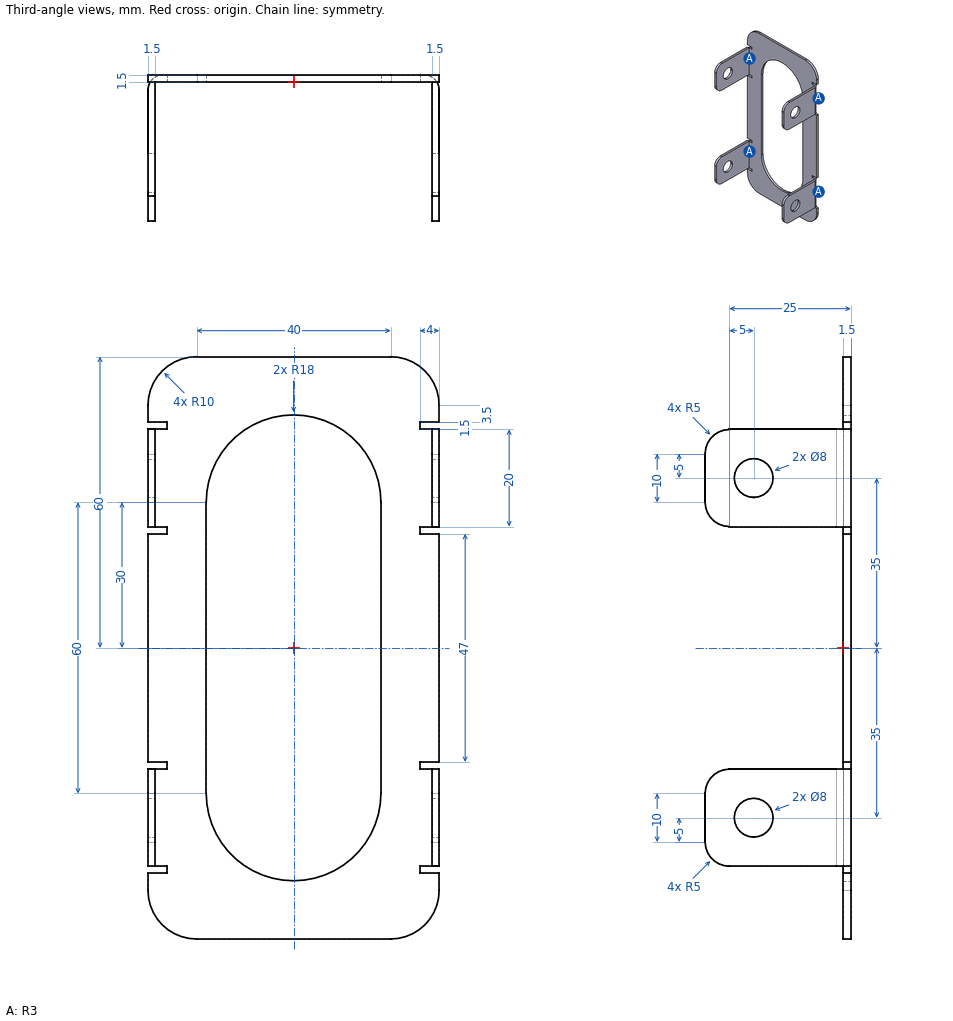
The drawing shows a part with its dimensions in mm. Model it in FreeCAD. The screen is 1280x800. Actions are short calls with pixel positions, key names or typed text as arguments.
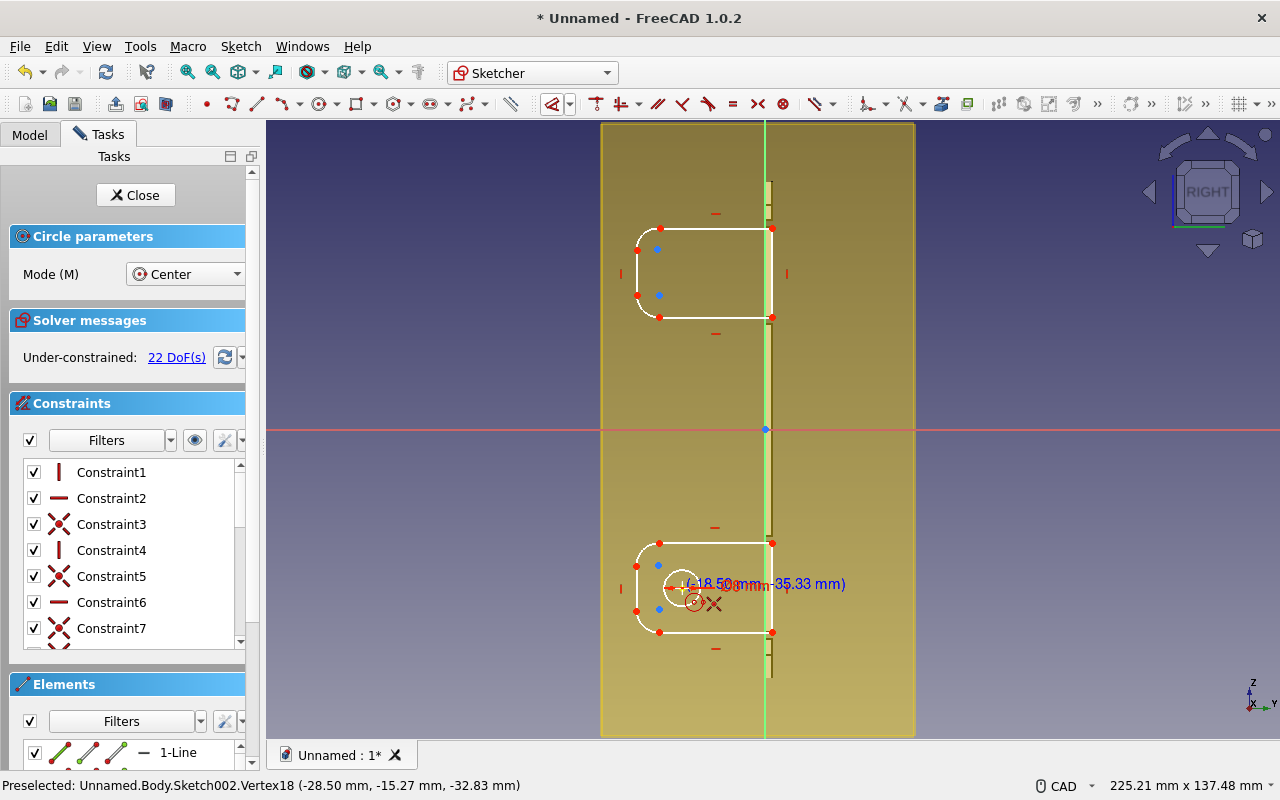
scroll(682, 272, up, 2)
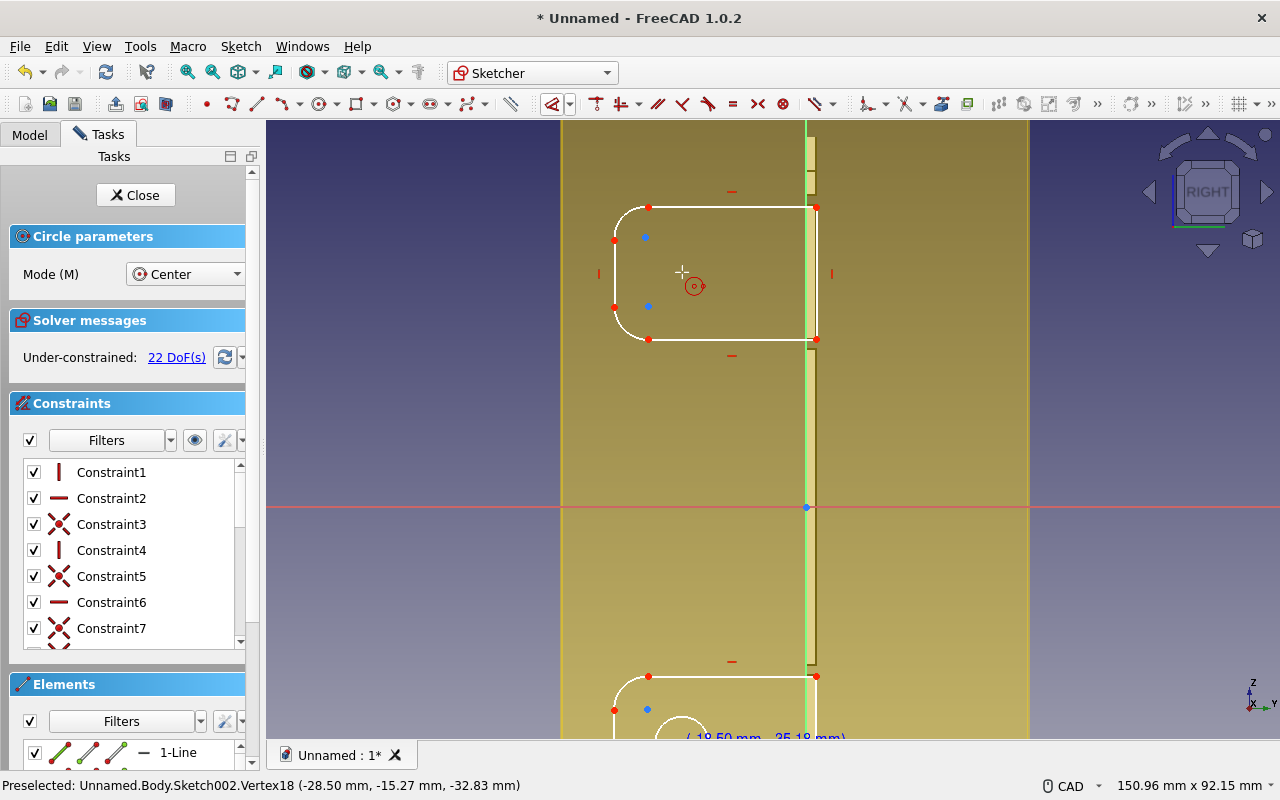
click(682, 272)
move(701, 253)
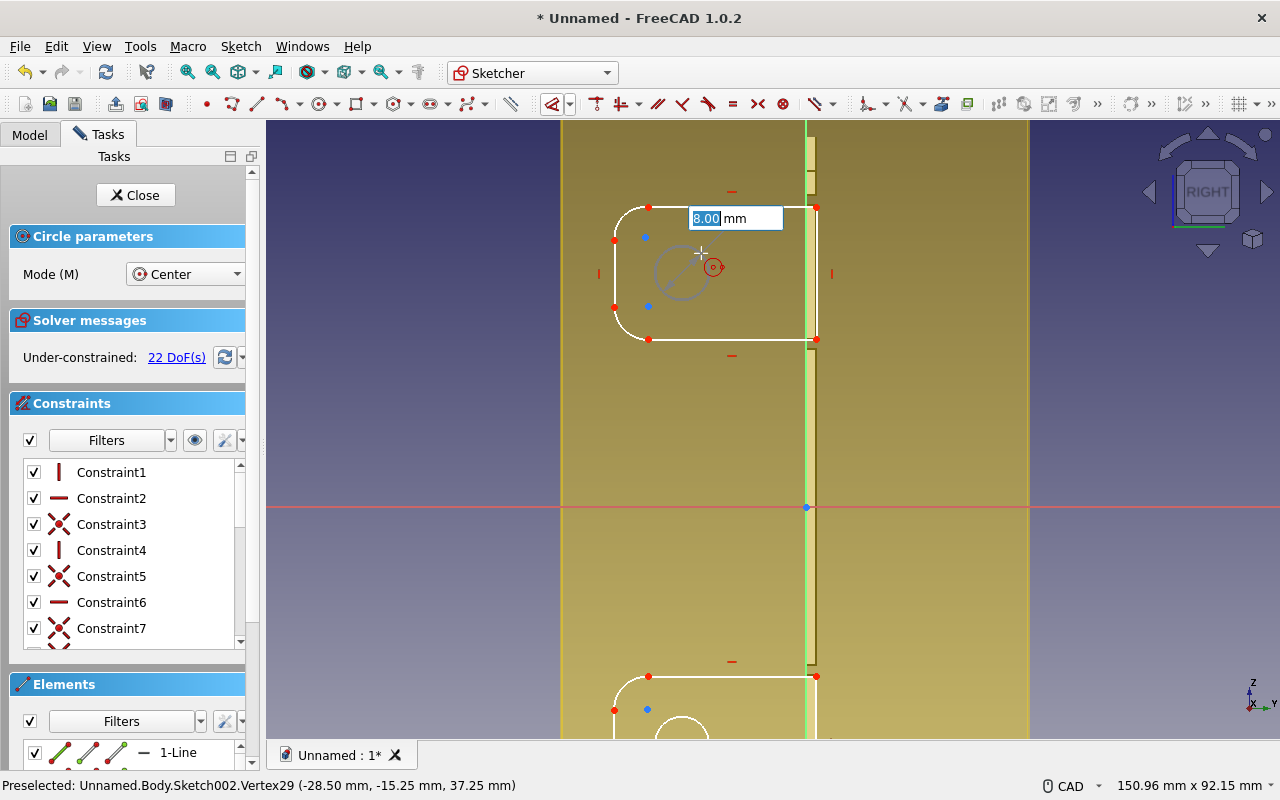
text(8)
key(Return)
key(Escape)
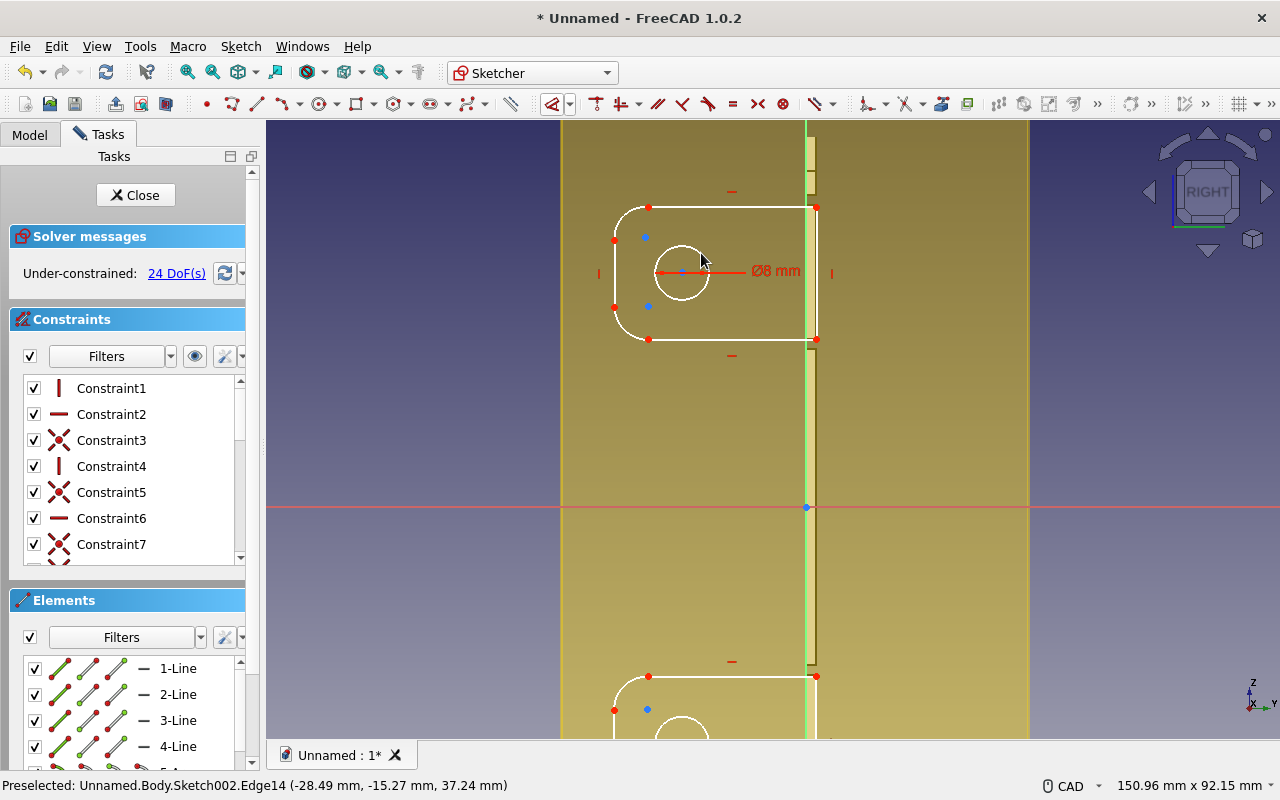
scroll(682, 271, down, 2)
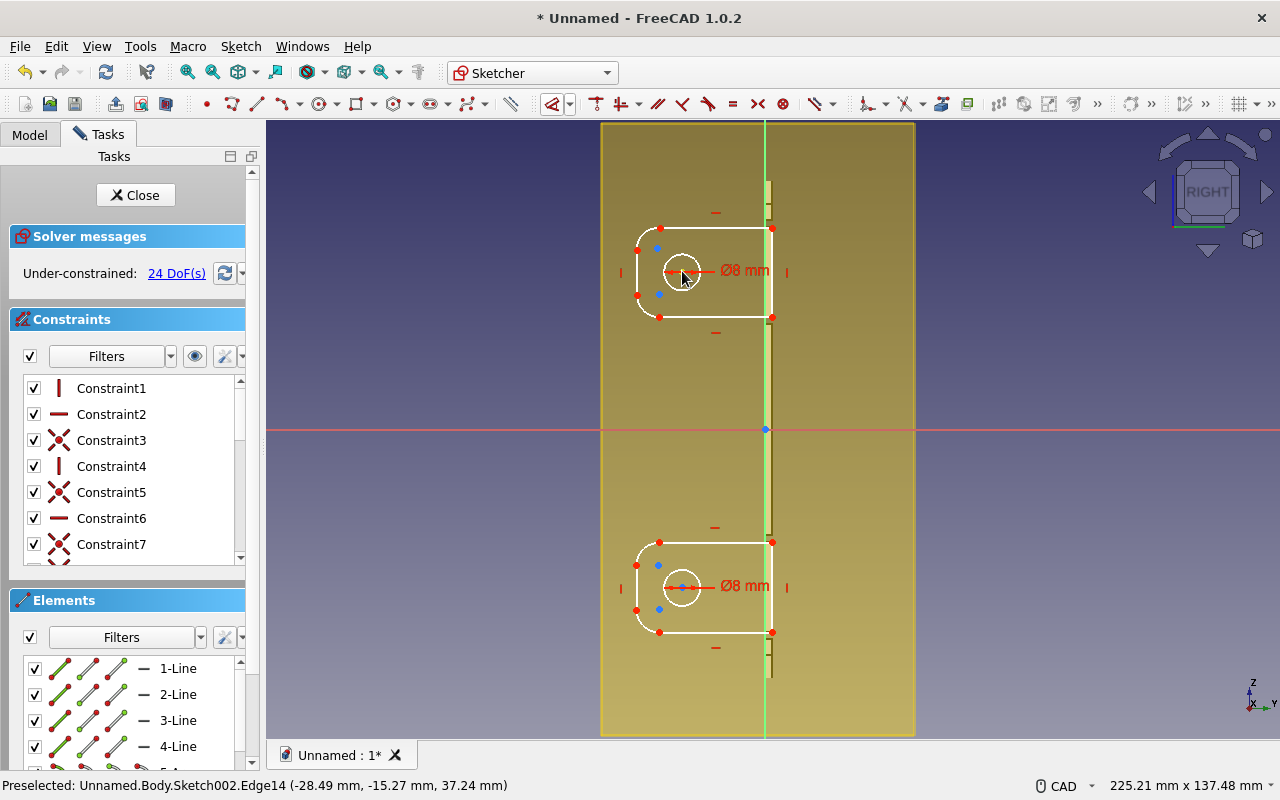
click(637, 597)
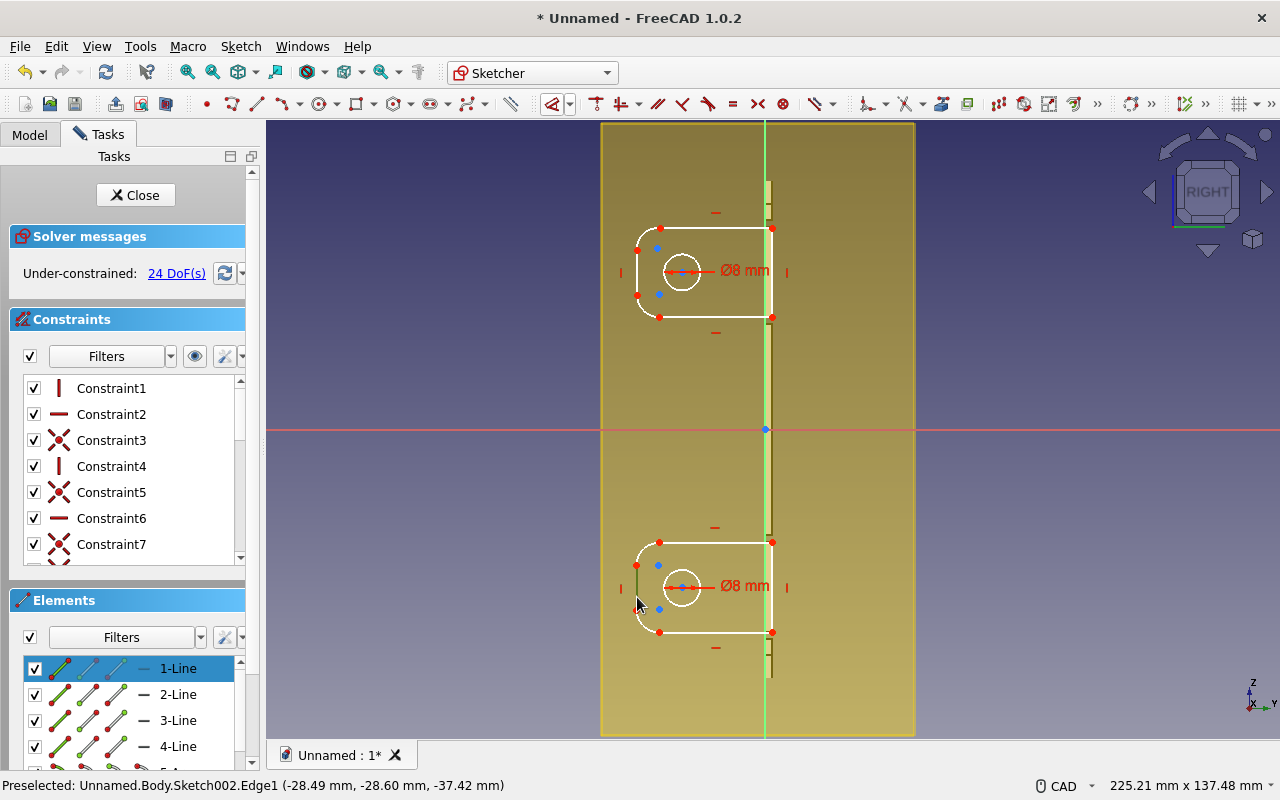
scroll(649, 545, up, 2)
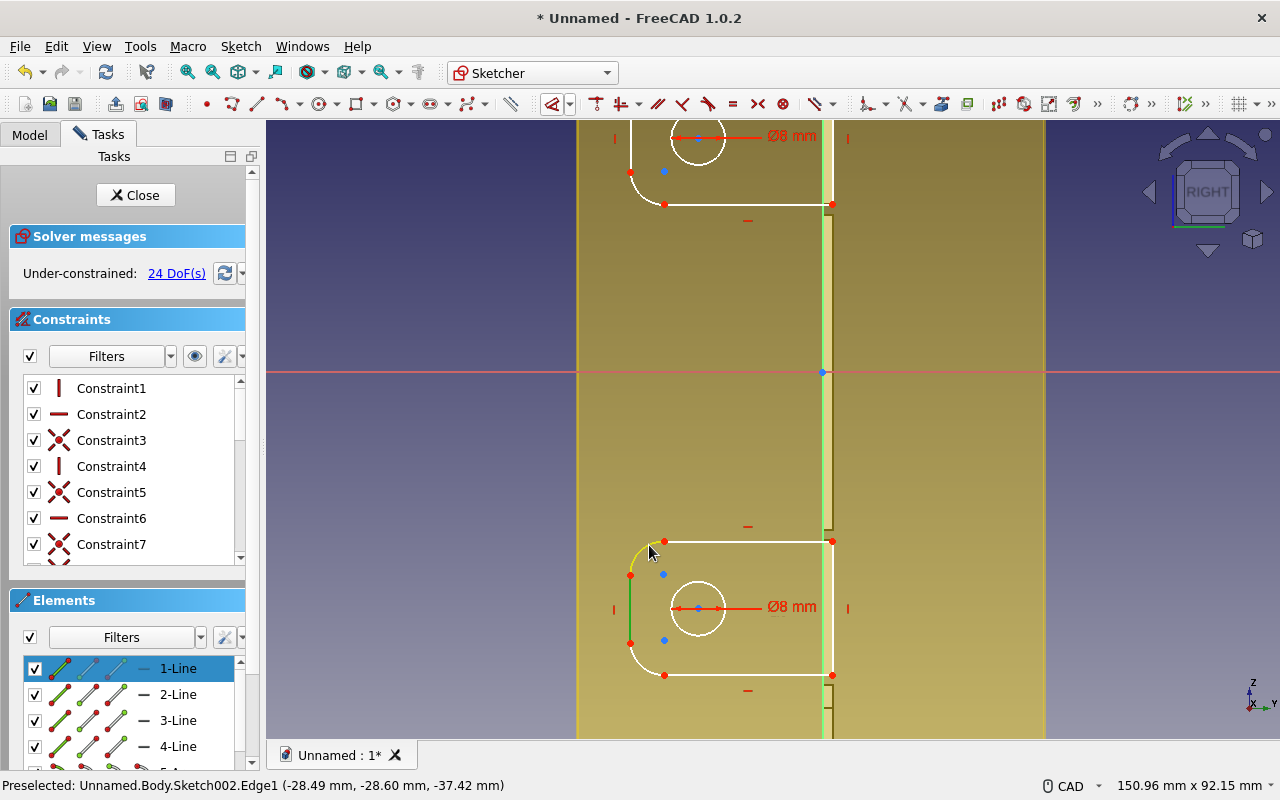
click(649, 545)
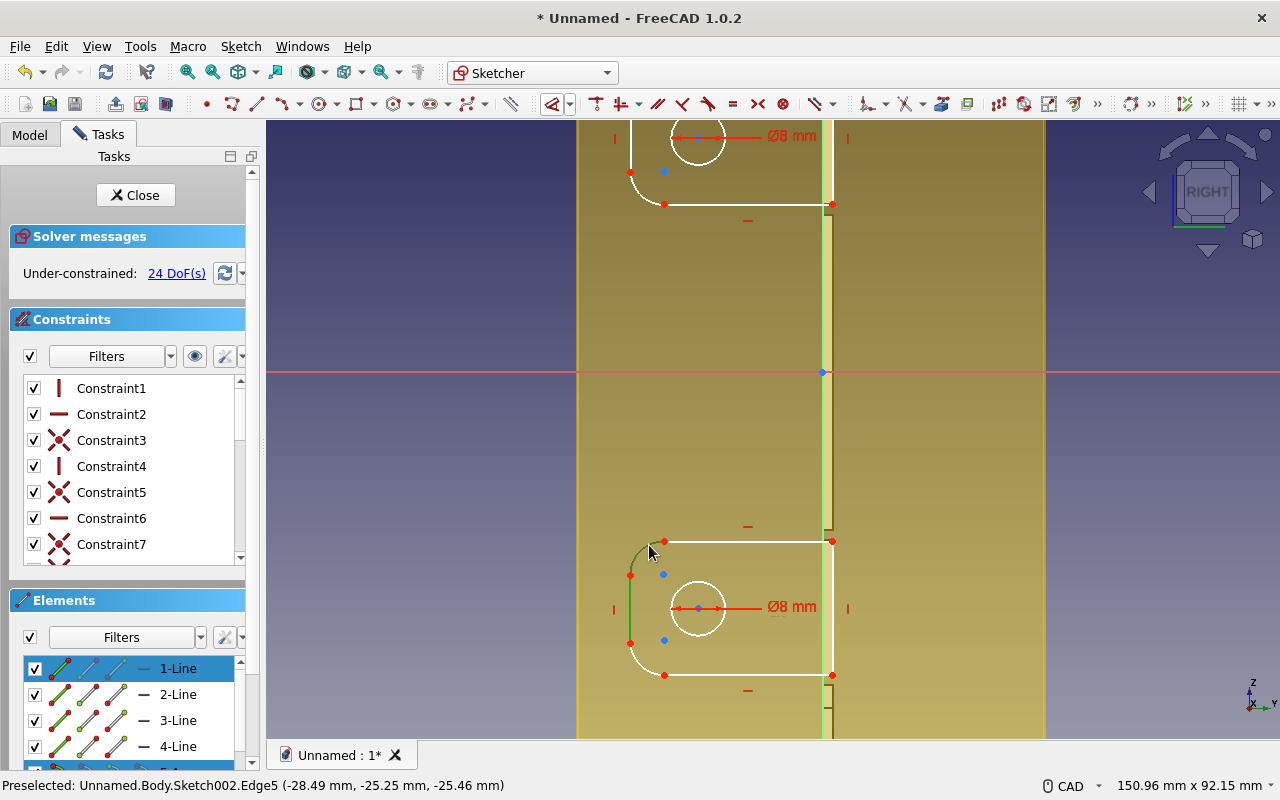
key(t)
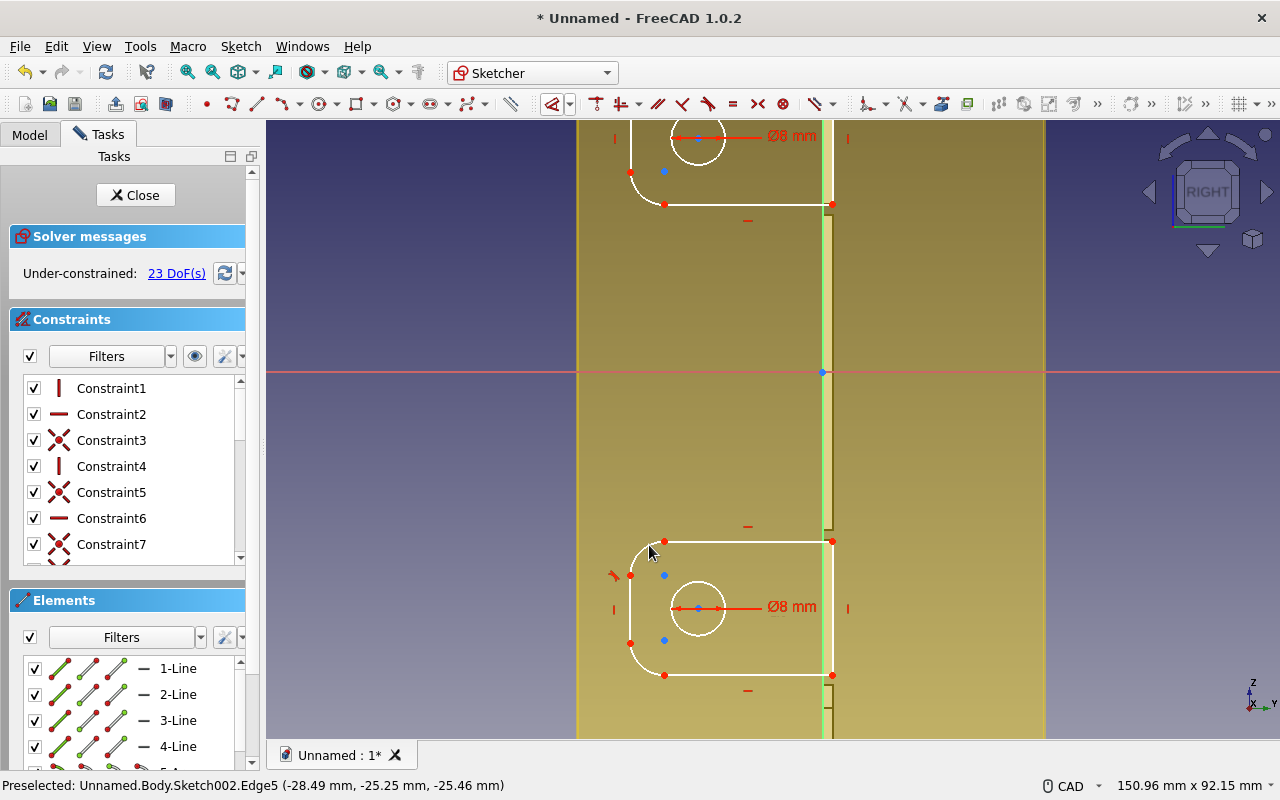
click(630, 623)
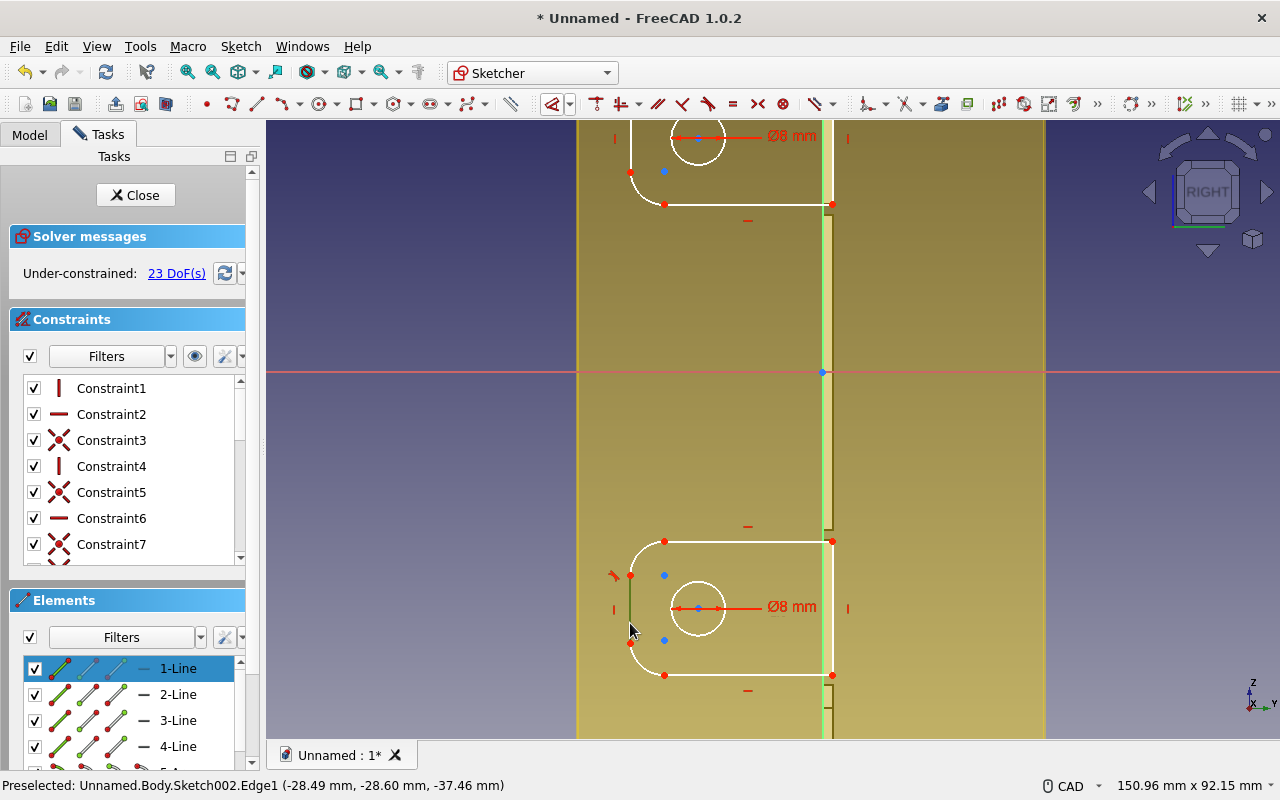
click(635, 658)